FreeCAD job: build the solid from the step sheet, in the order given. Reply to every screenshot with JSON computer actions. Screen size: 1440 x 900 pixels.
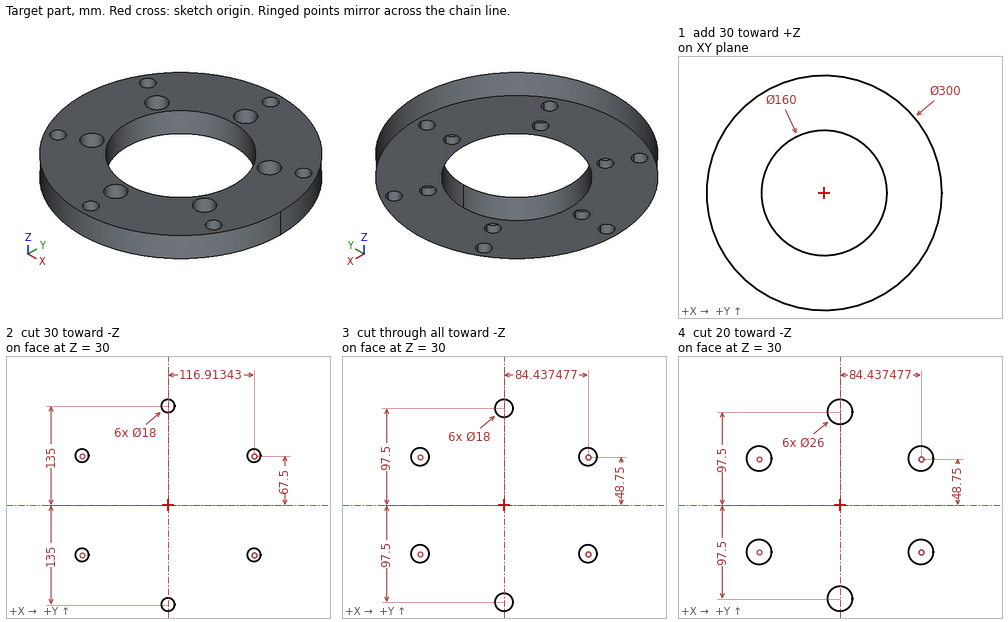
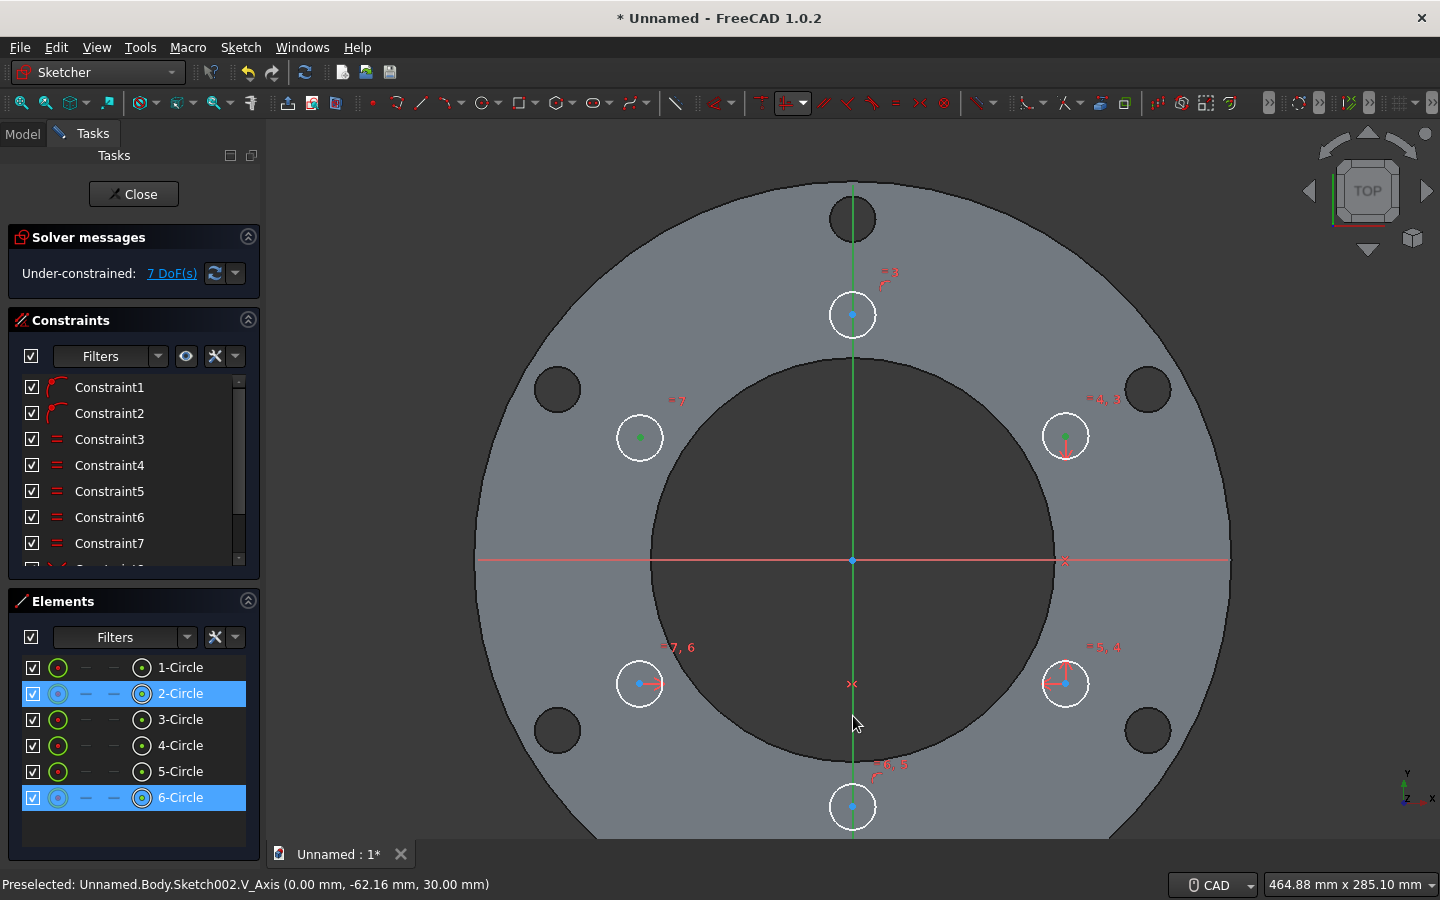
{"action": "key", "text": "s"}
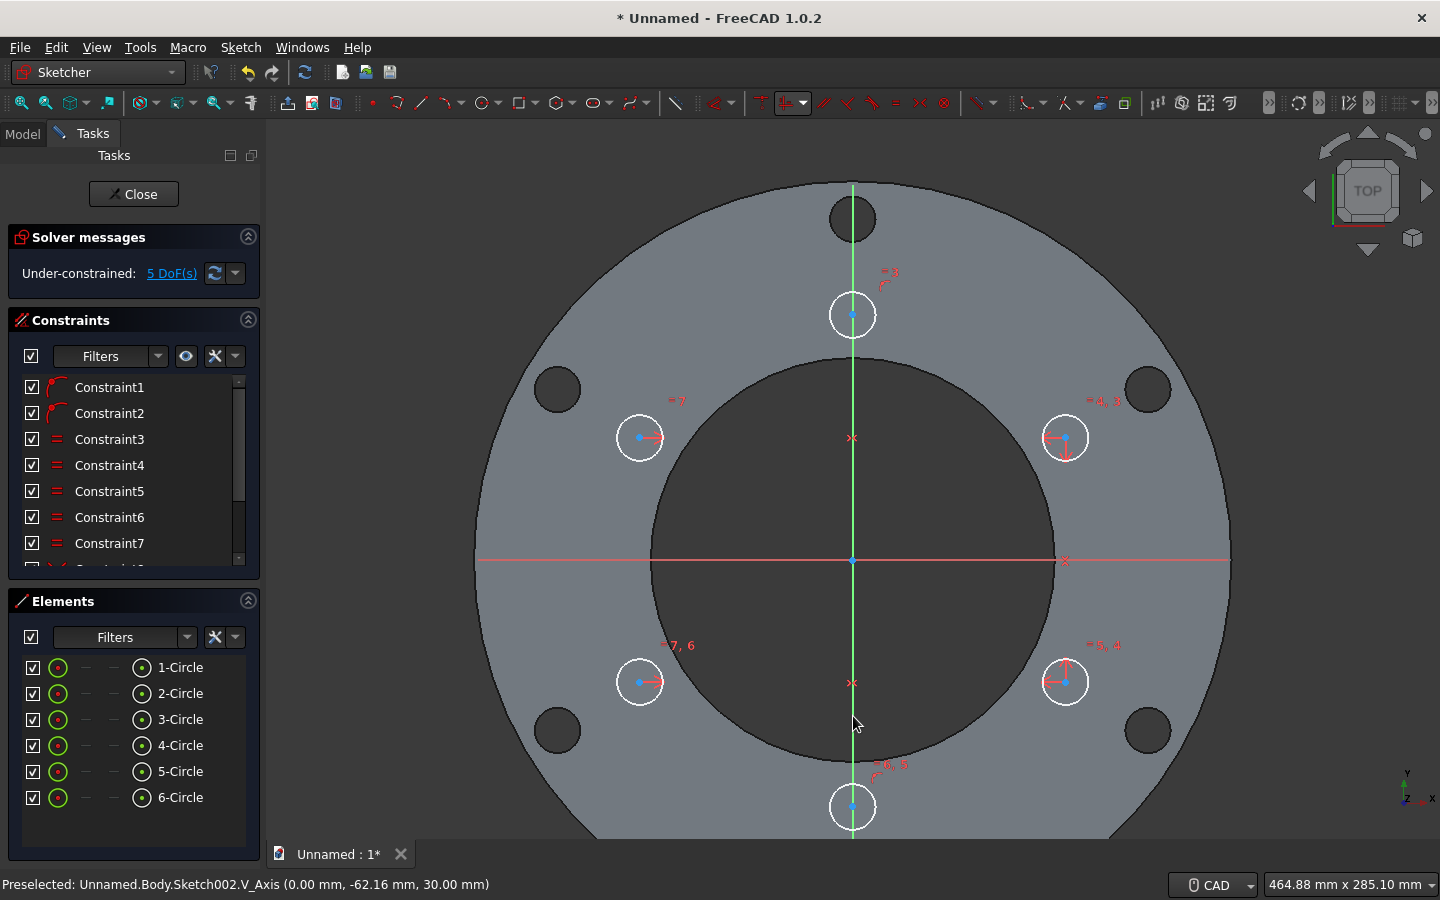
{"action": "left_click", "coordinate": [869, 299]}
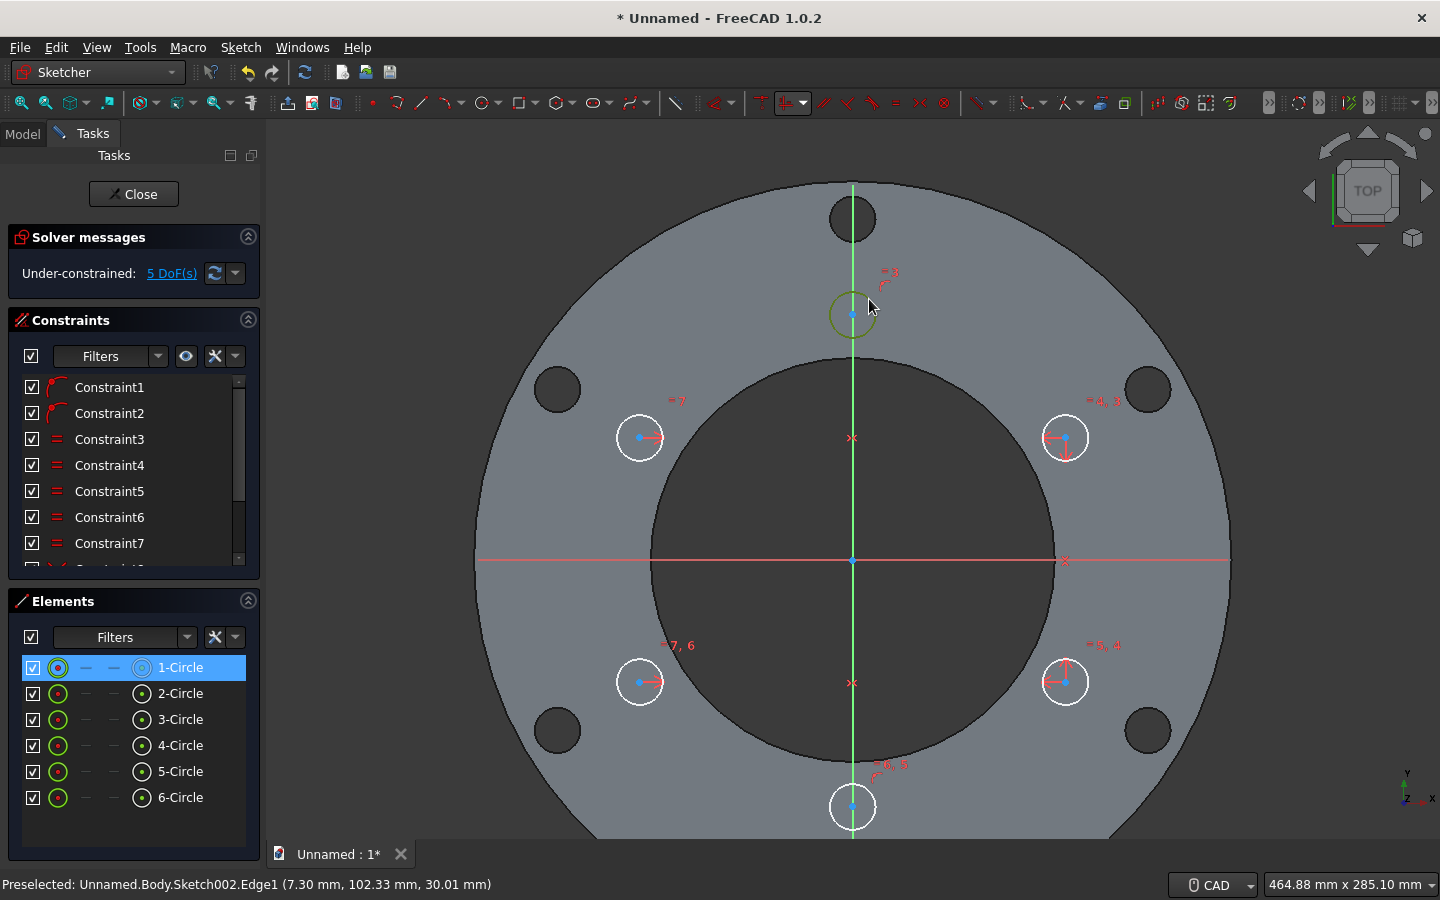
{"action": "key", "text": "k o"}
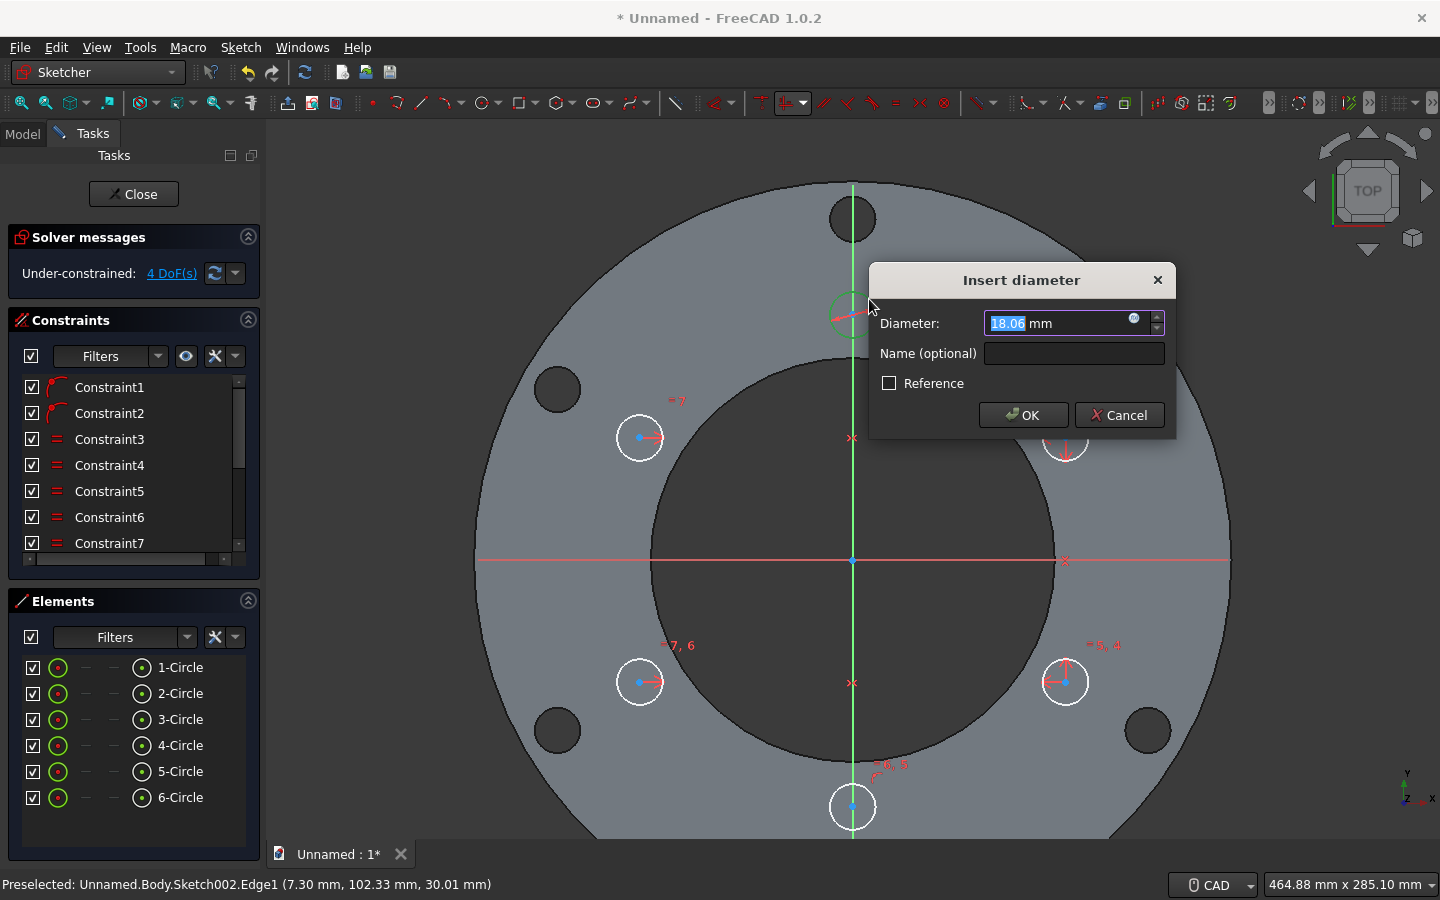
{"action": "type", "text": "18"}
{"action": "key", "text": "Return"}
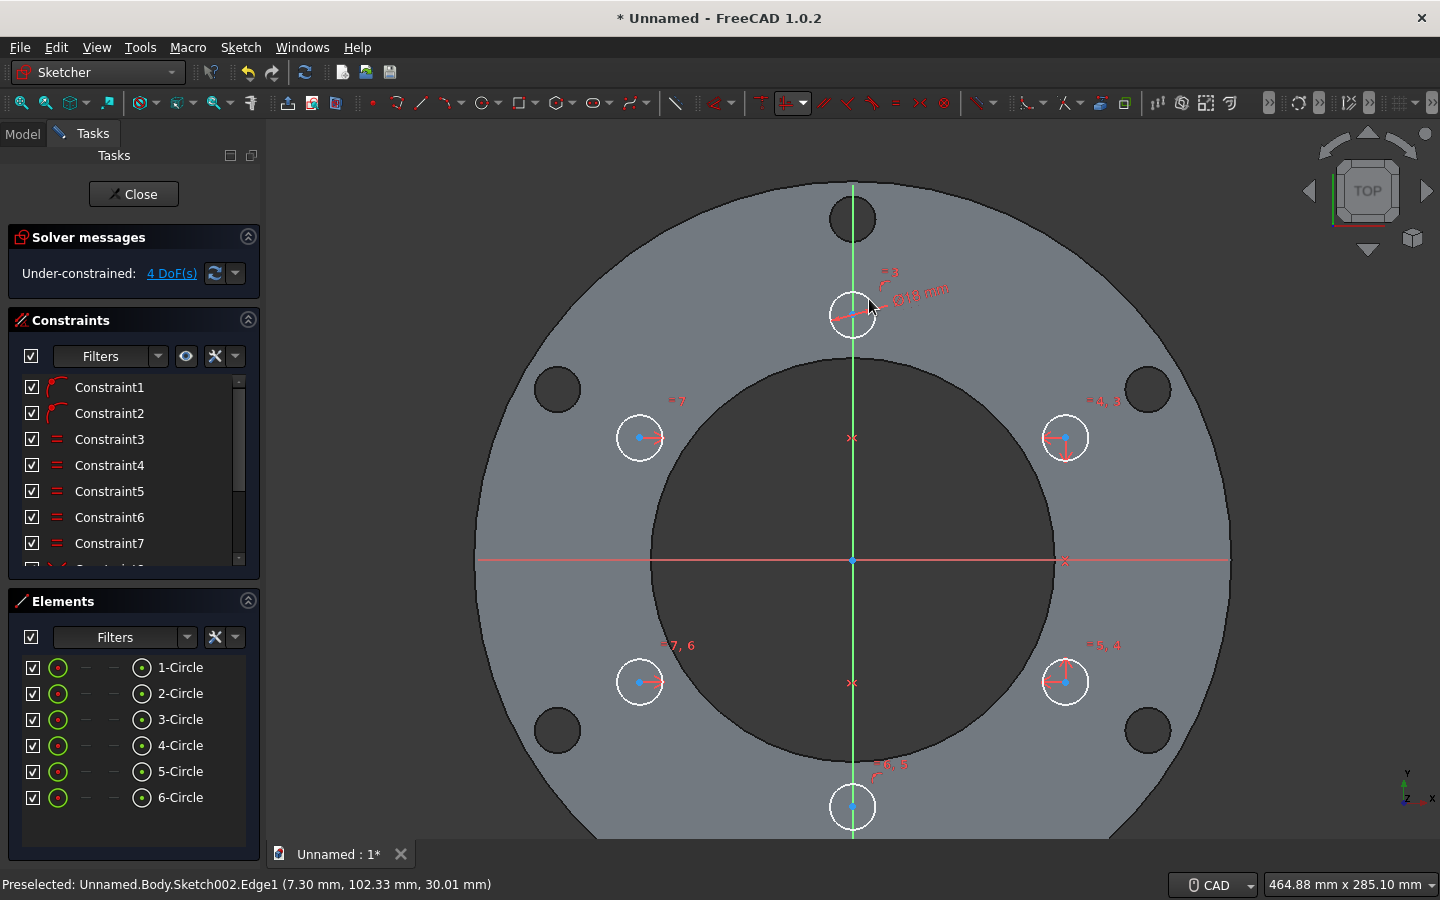
{"action": "left_click", "coordinate": [853, 315]}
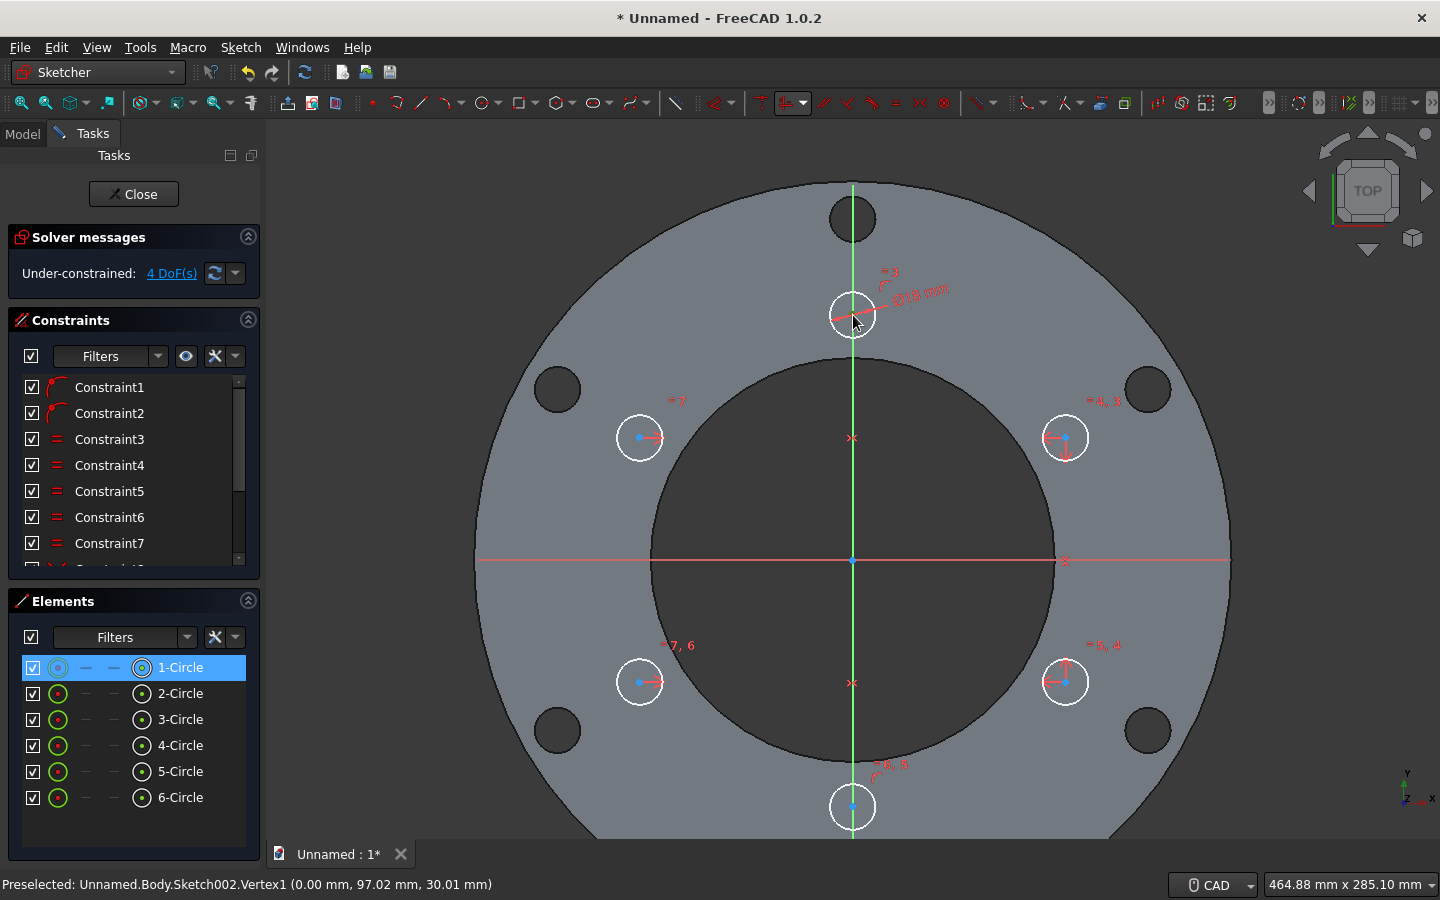
{"action": "key", "text": "i"}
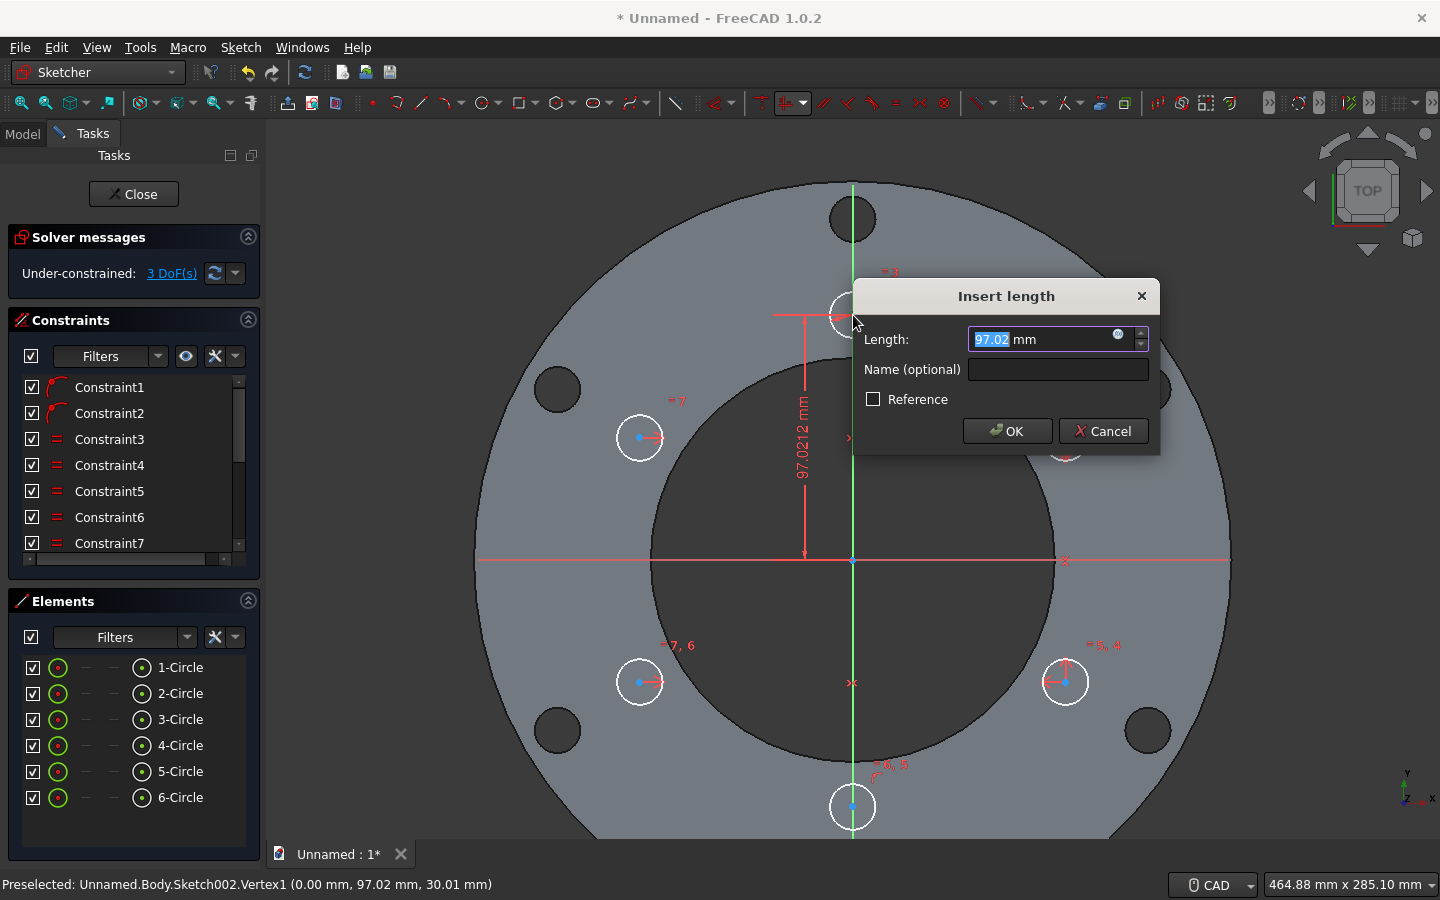
{"action": "type", "text": "97.5"}
{"action": "key", "text": "Return"}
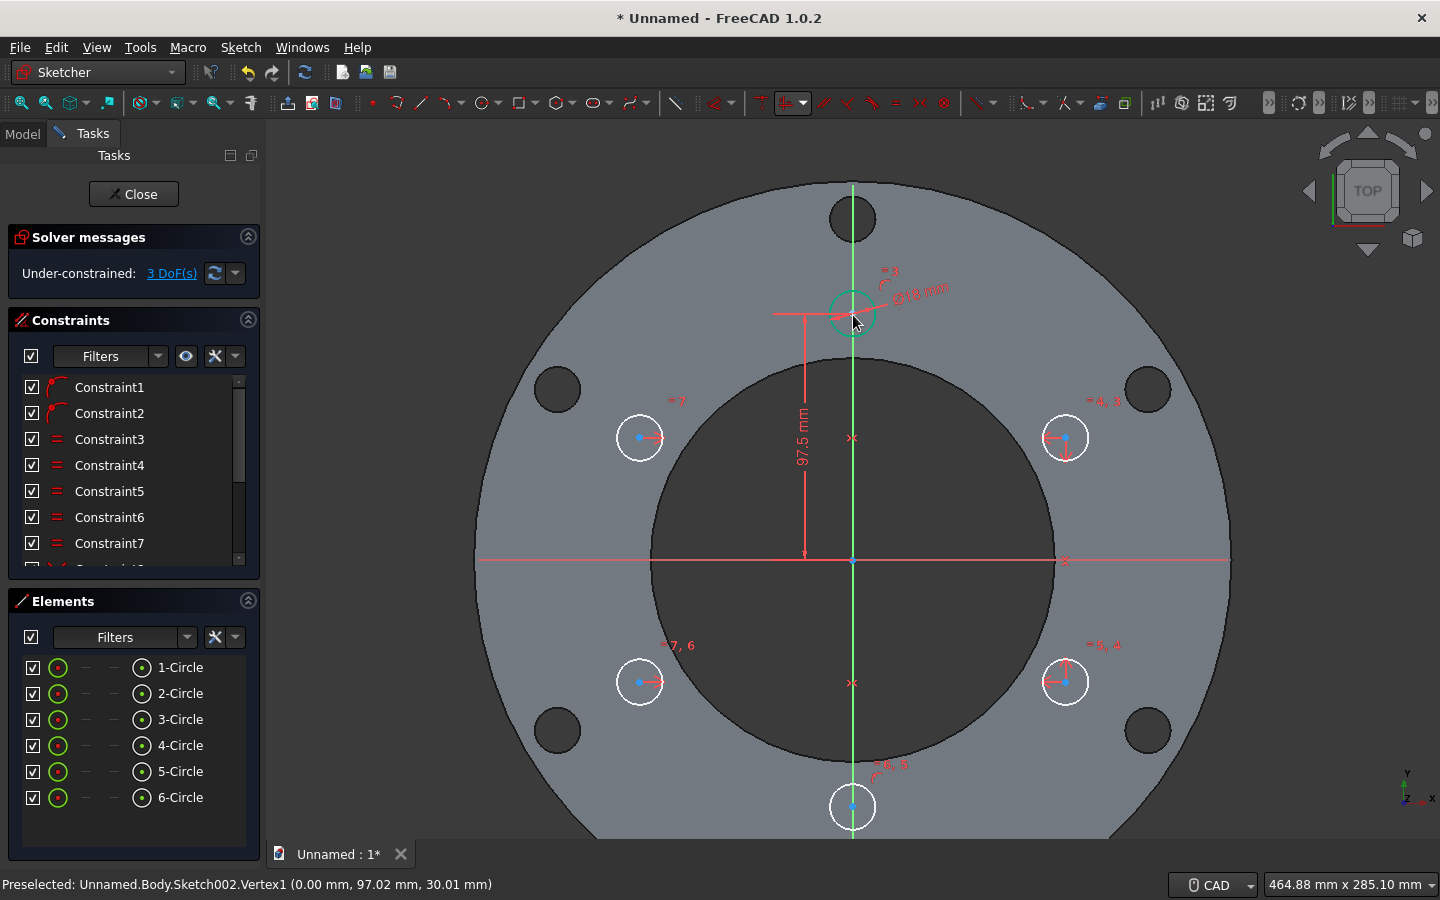
{"action": "left_click", "coordinate": [853, 807]}